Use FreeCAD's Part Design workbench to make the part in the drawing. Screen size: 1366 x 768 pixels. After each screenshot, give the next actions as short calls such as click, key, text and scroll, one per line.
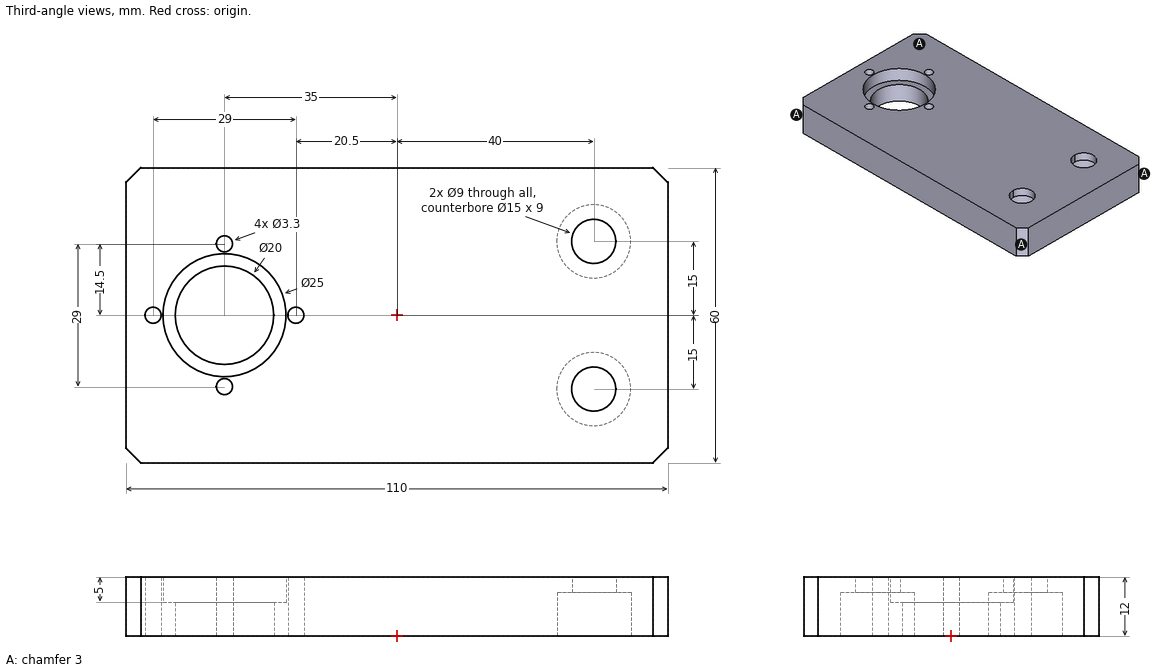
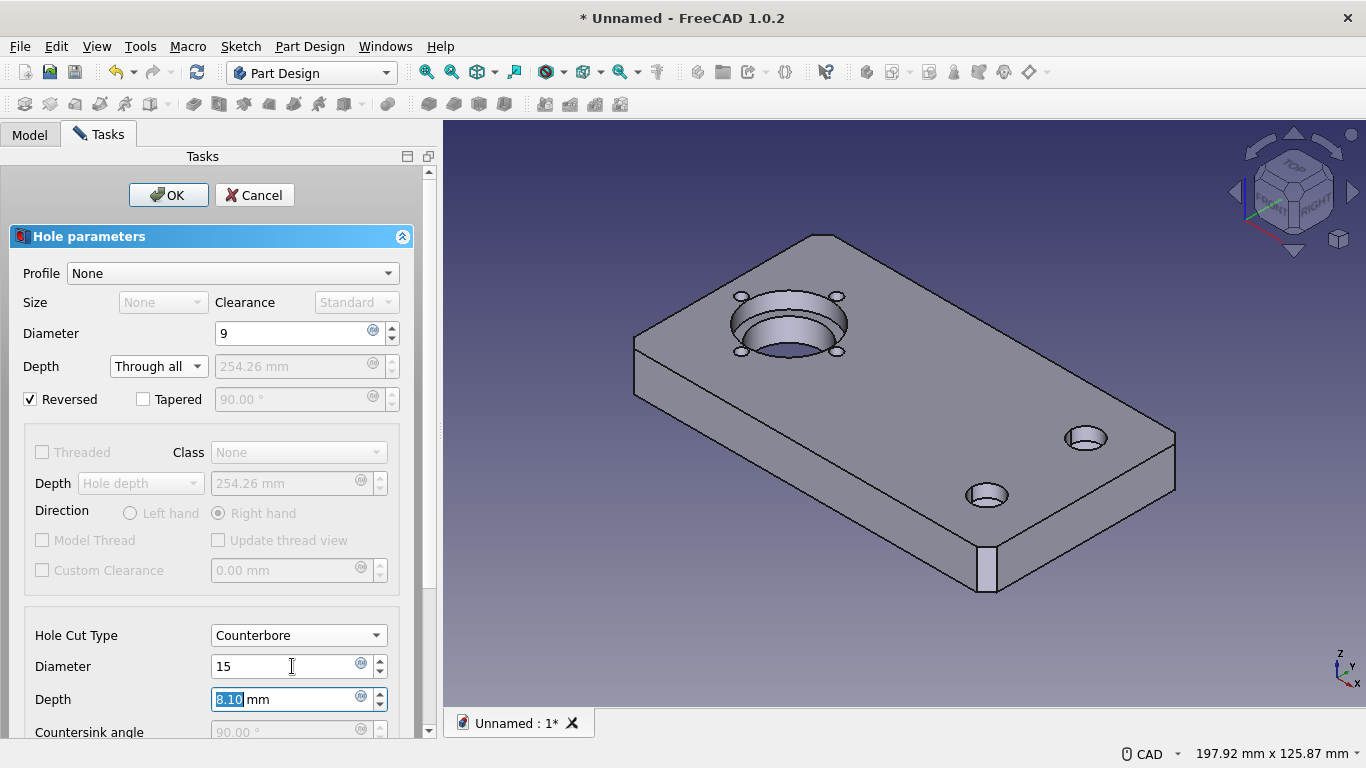
text(9)
key(Tab)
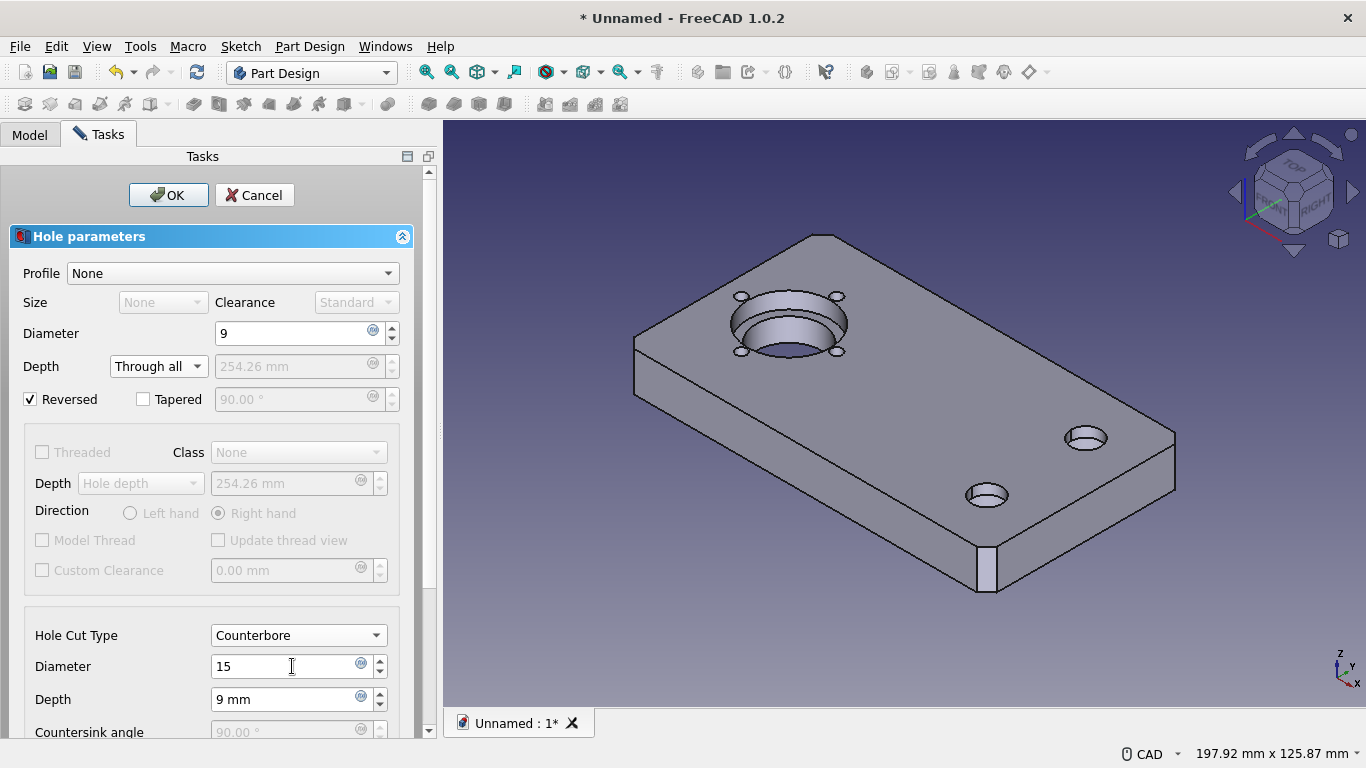
click(169, 195)